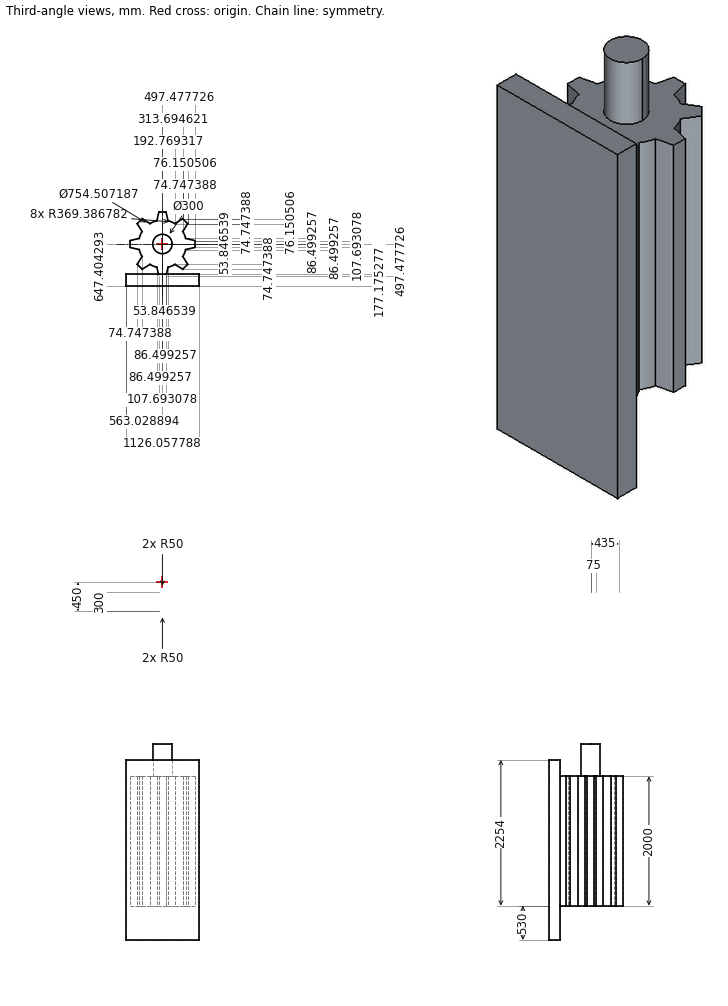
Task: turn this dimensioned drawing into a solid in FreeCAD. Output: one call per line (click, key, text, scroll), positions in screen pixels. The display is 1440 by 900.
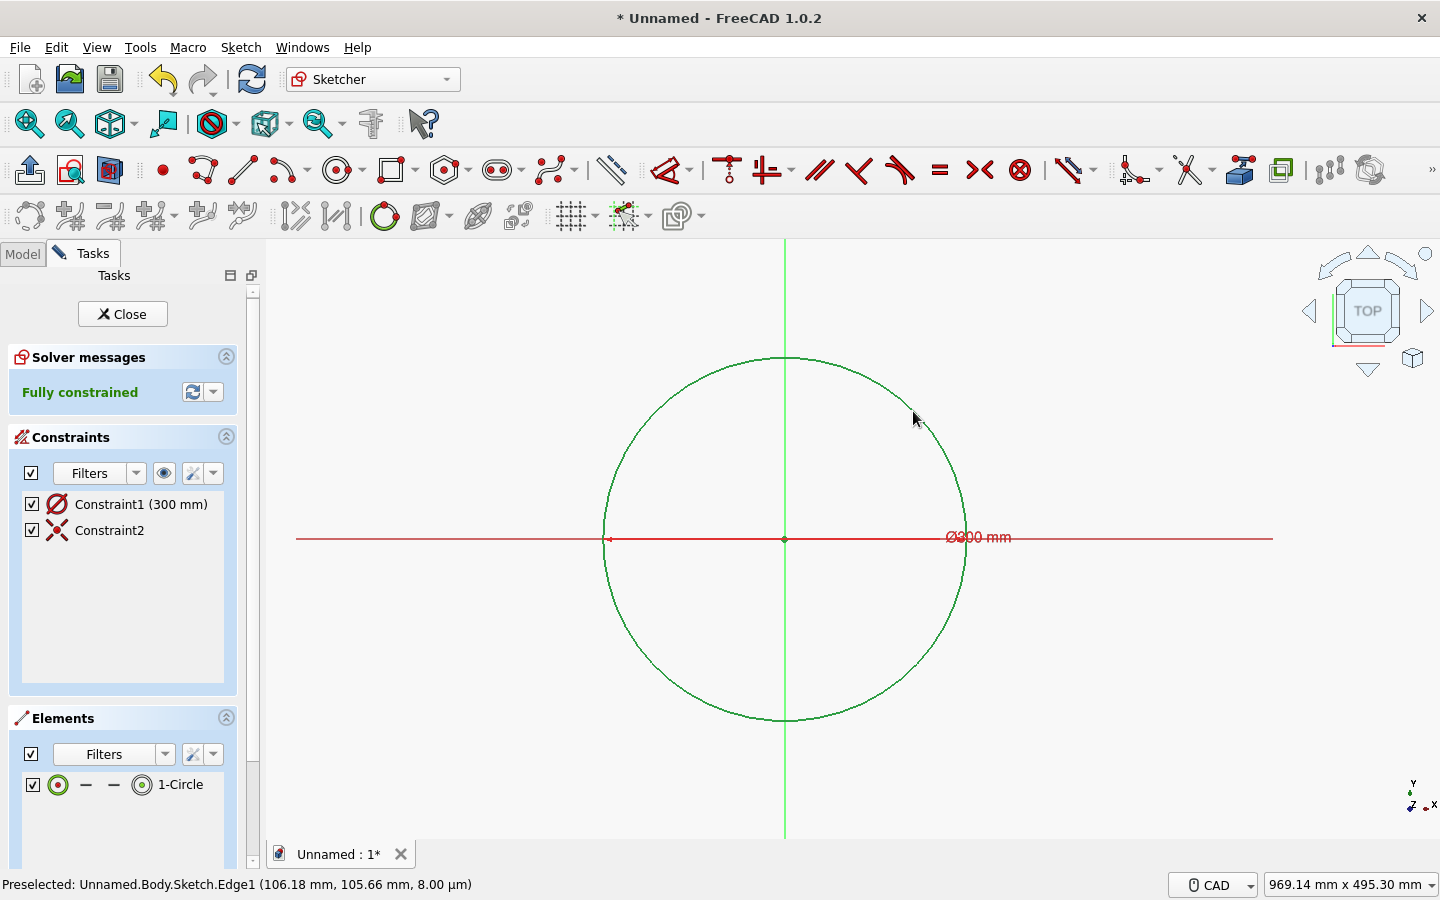
click(123, 314)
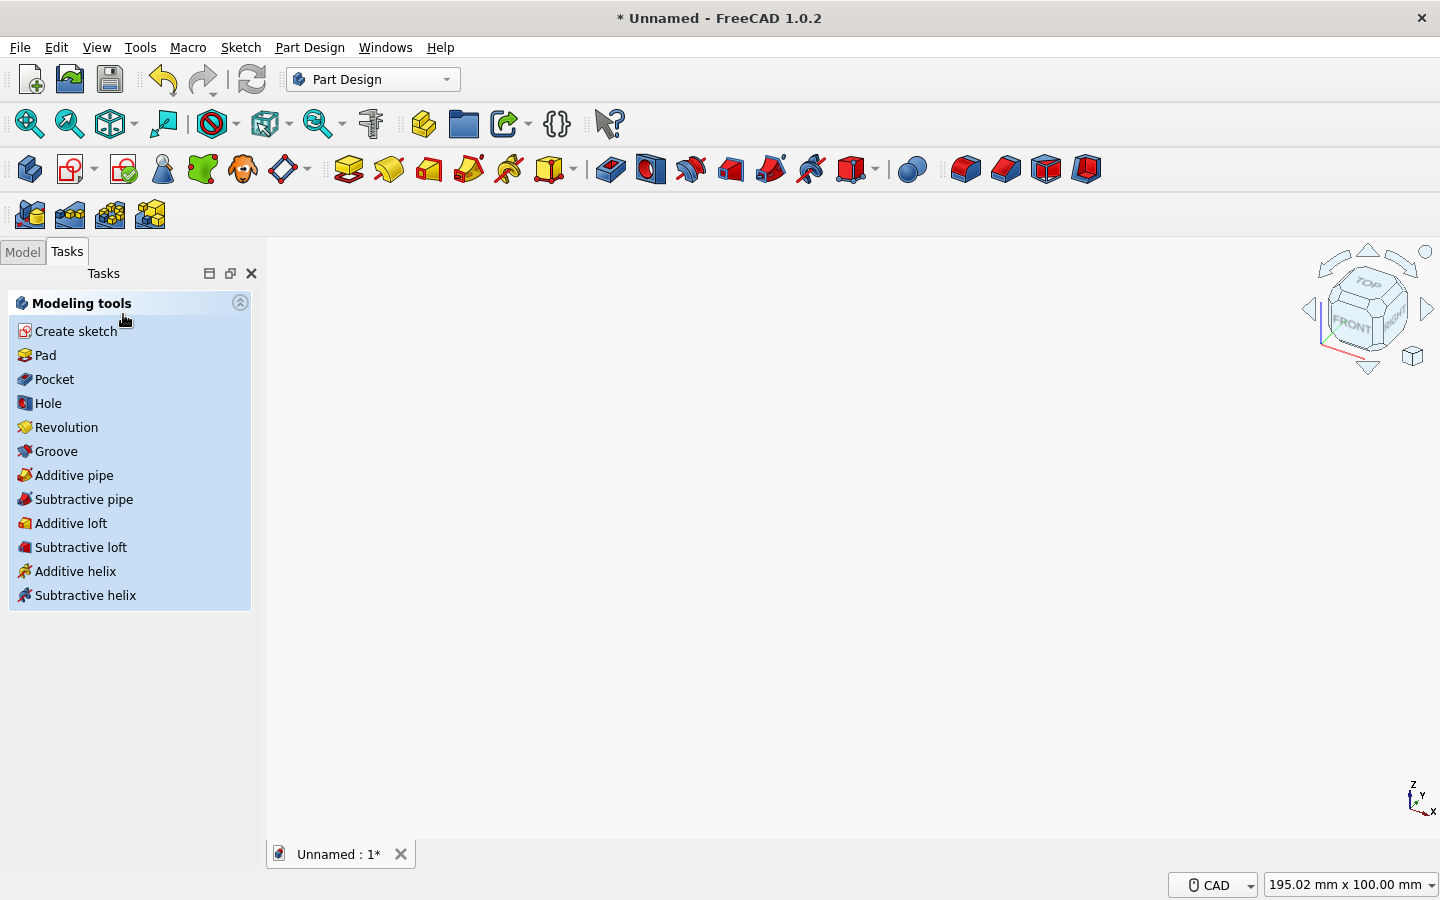
click(350, 170)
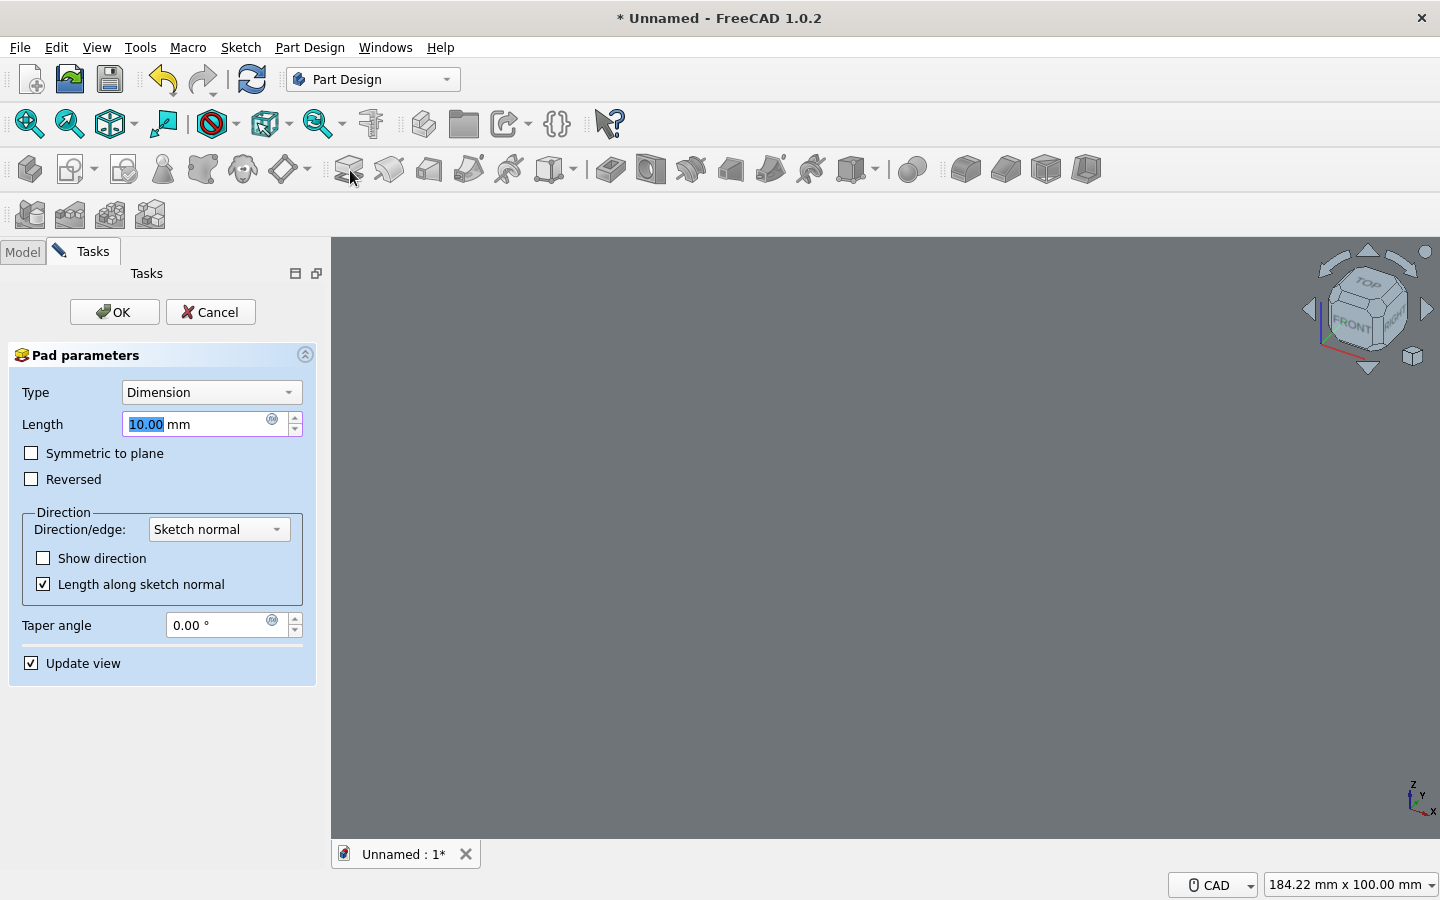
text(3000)
key(Tab)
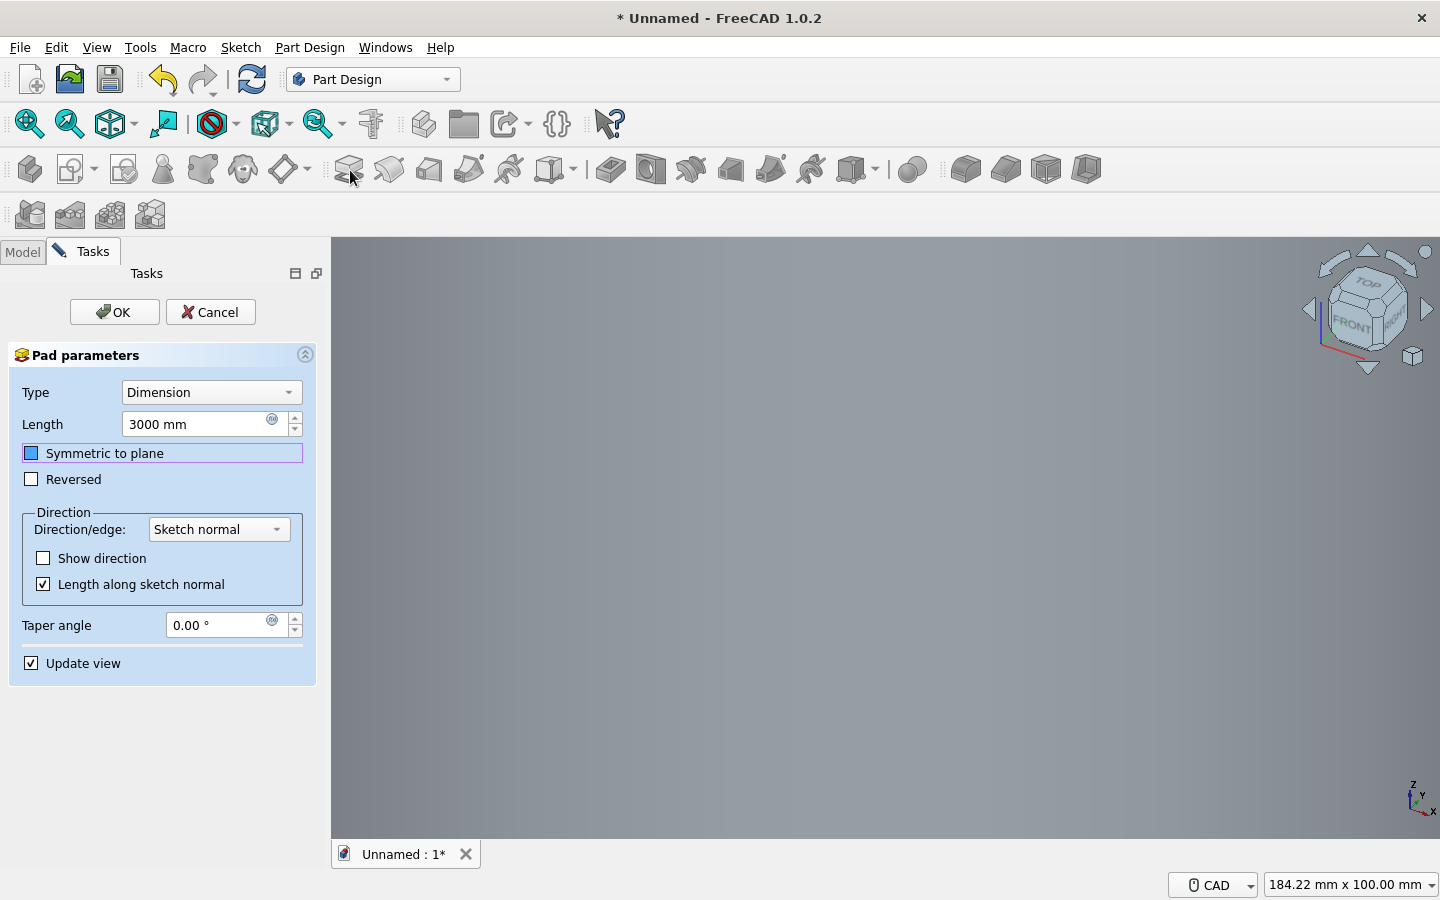
click(30, 479)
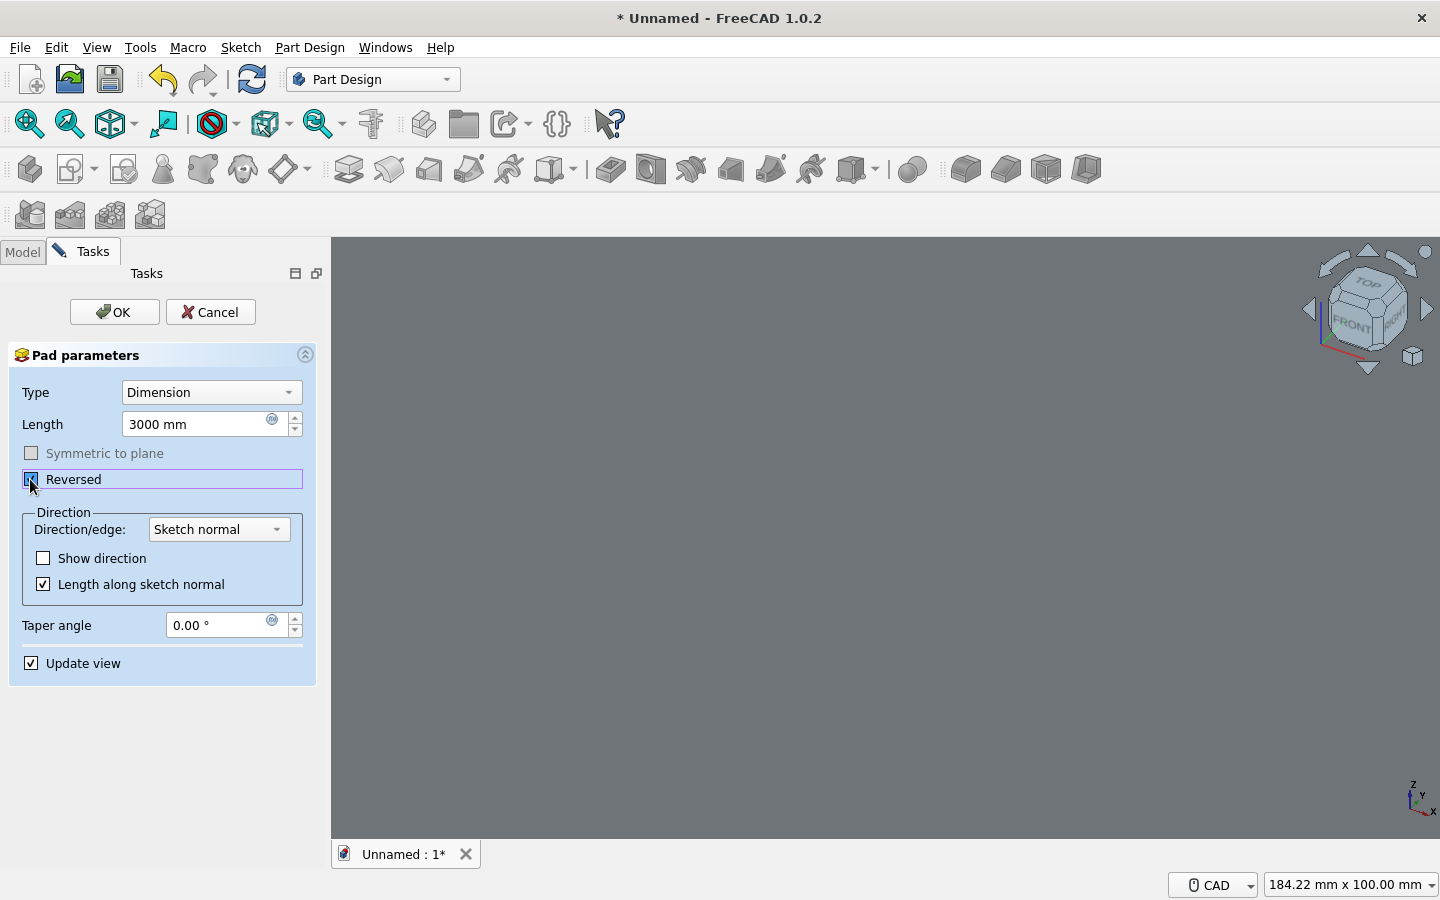
click(115, 312)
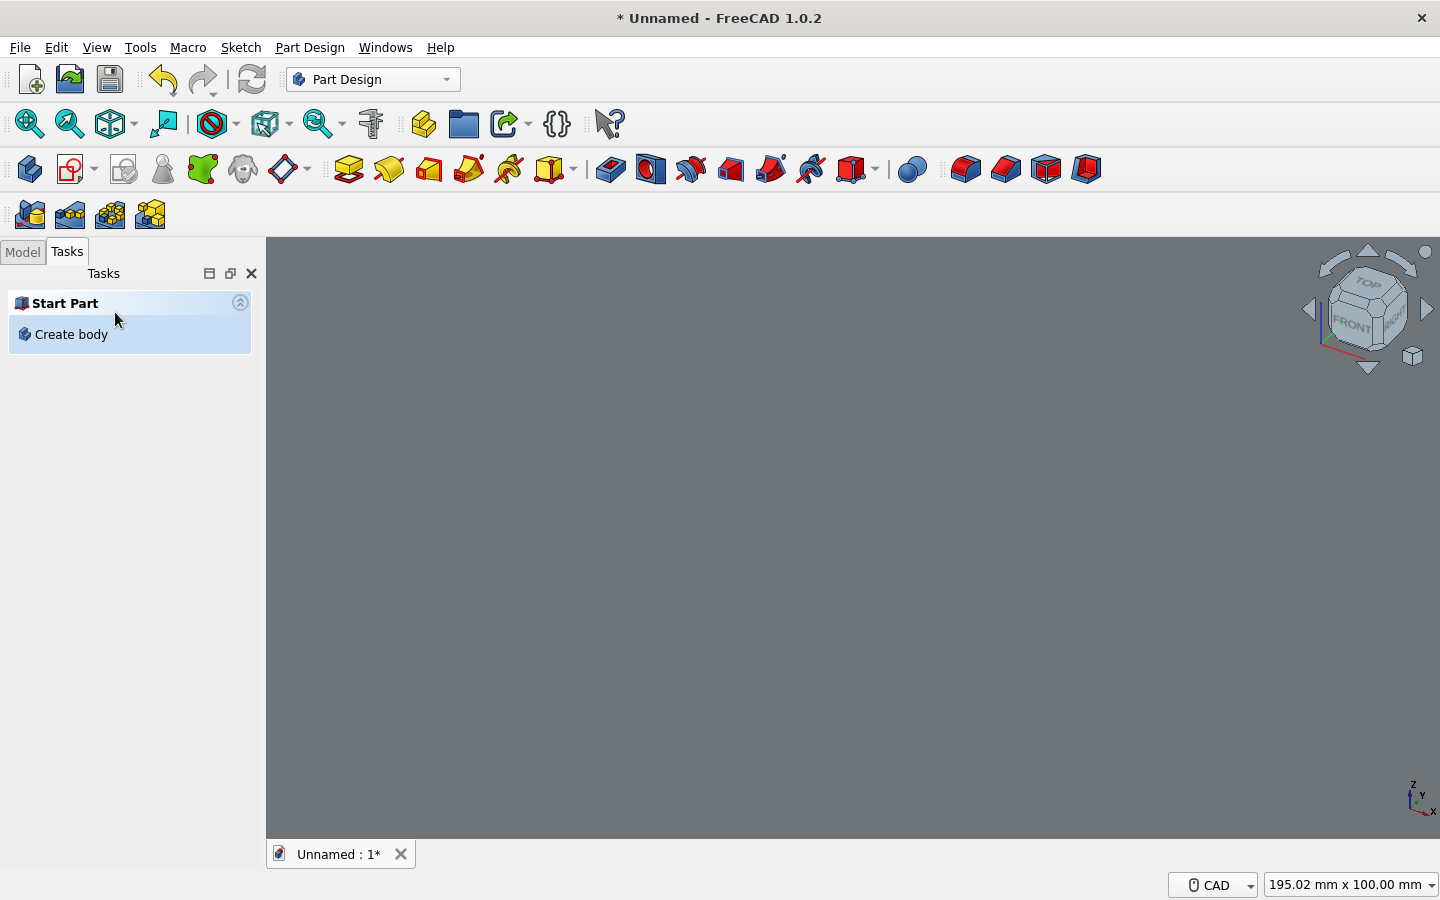
click(30, 124)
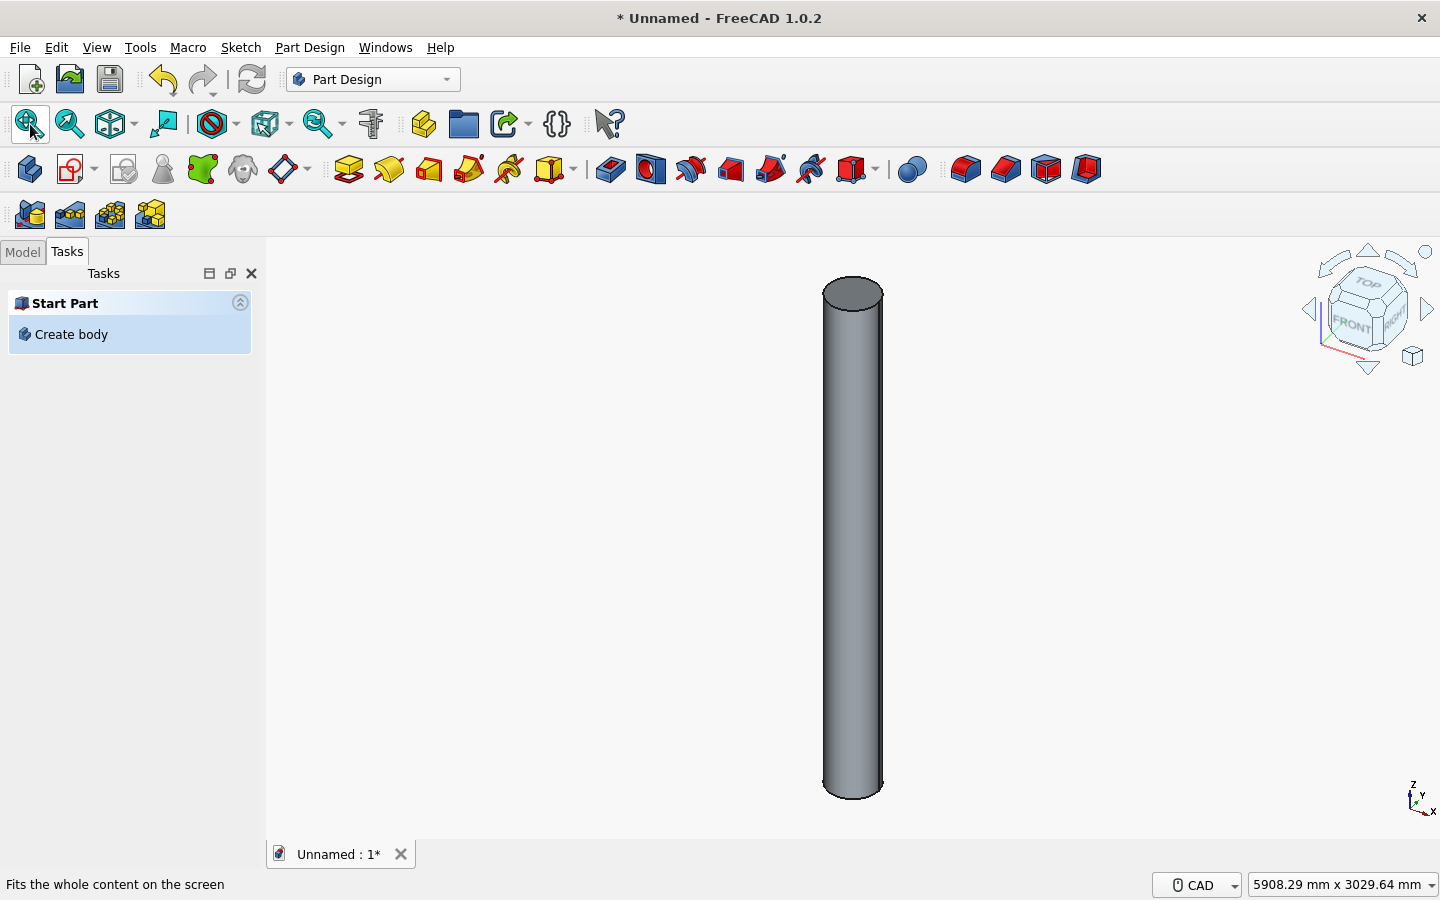
click(70, 170)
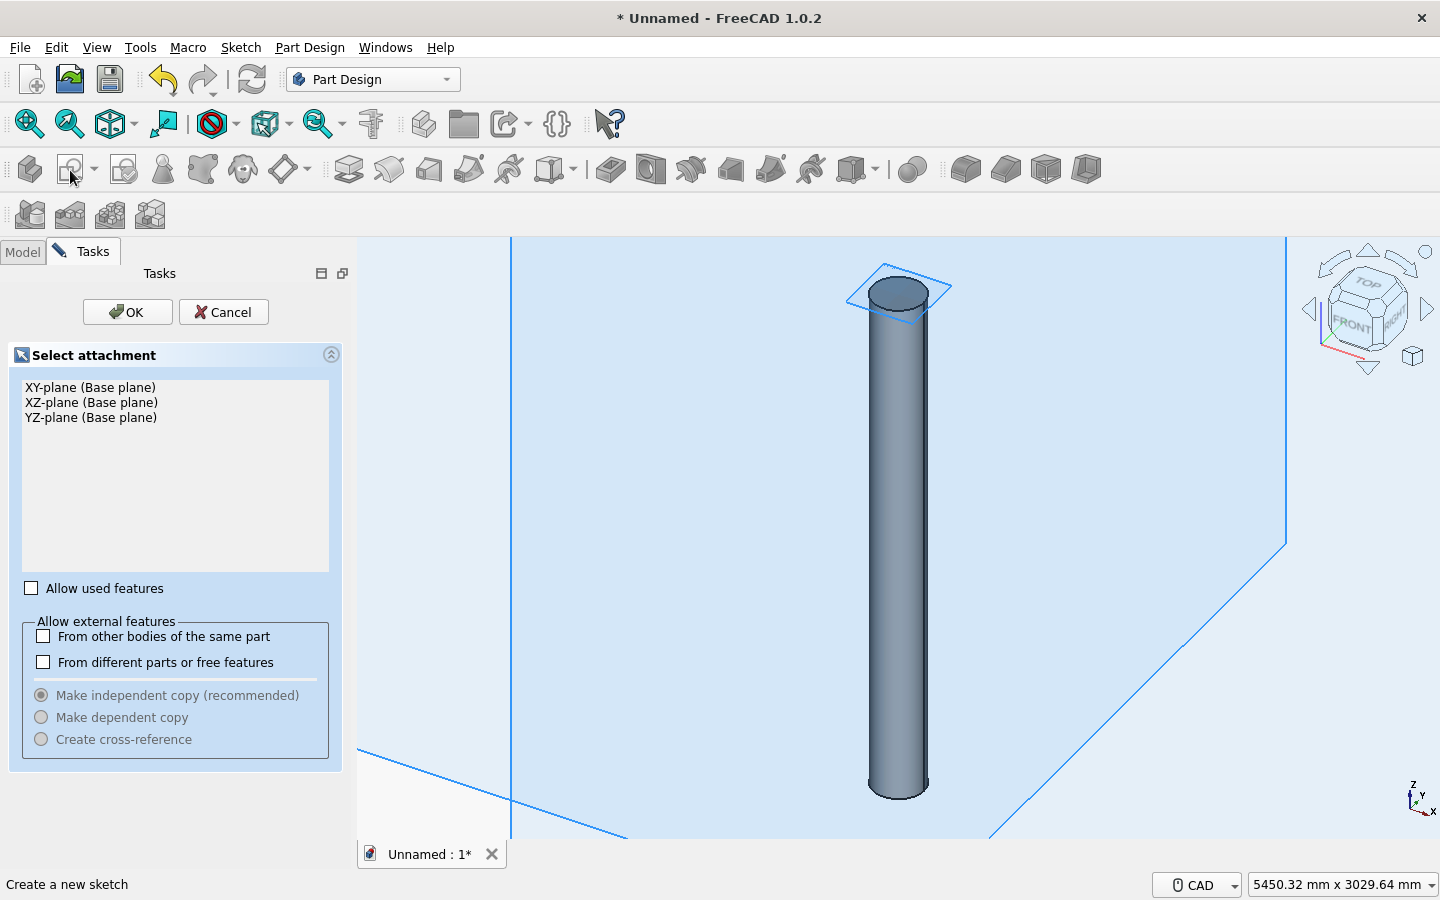
click(82, 402)